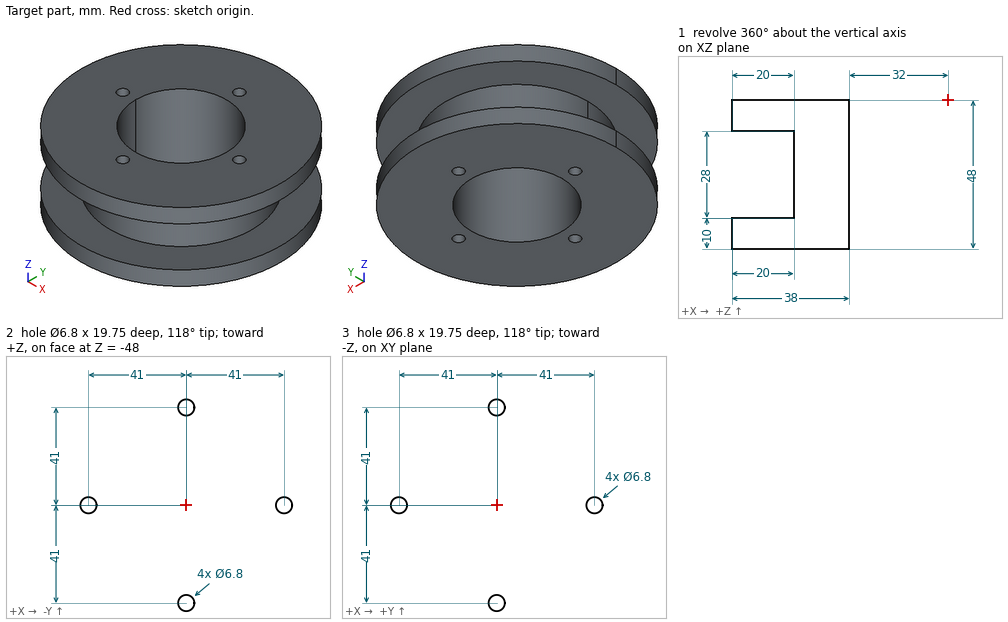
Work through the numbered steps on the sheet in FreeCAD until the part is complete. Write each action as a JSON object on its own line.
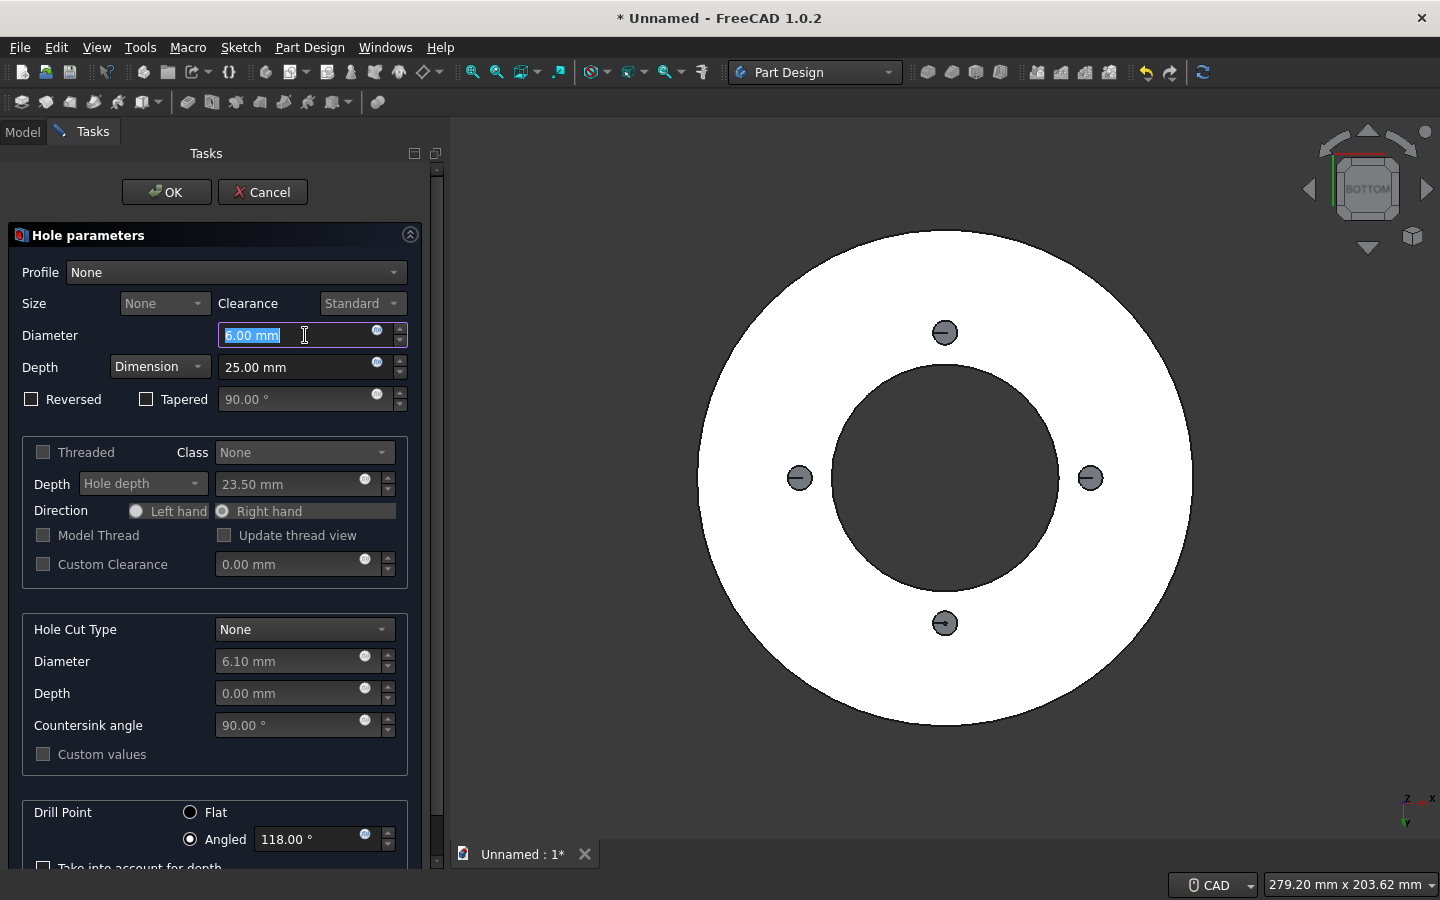
{"action": "type", "text": "6.8"}
{"action": "key", "text": "Tab"}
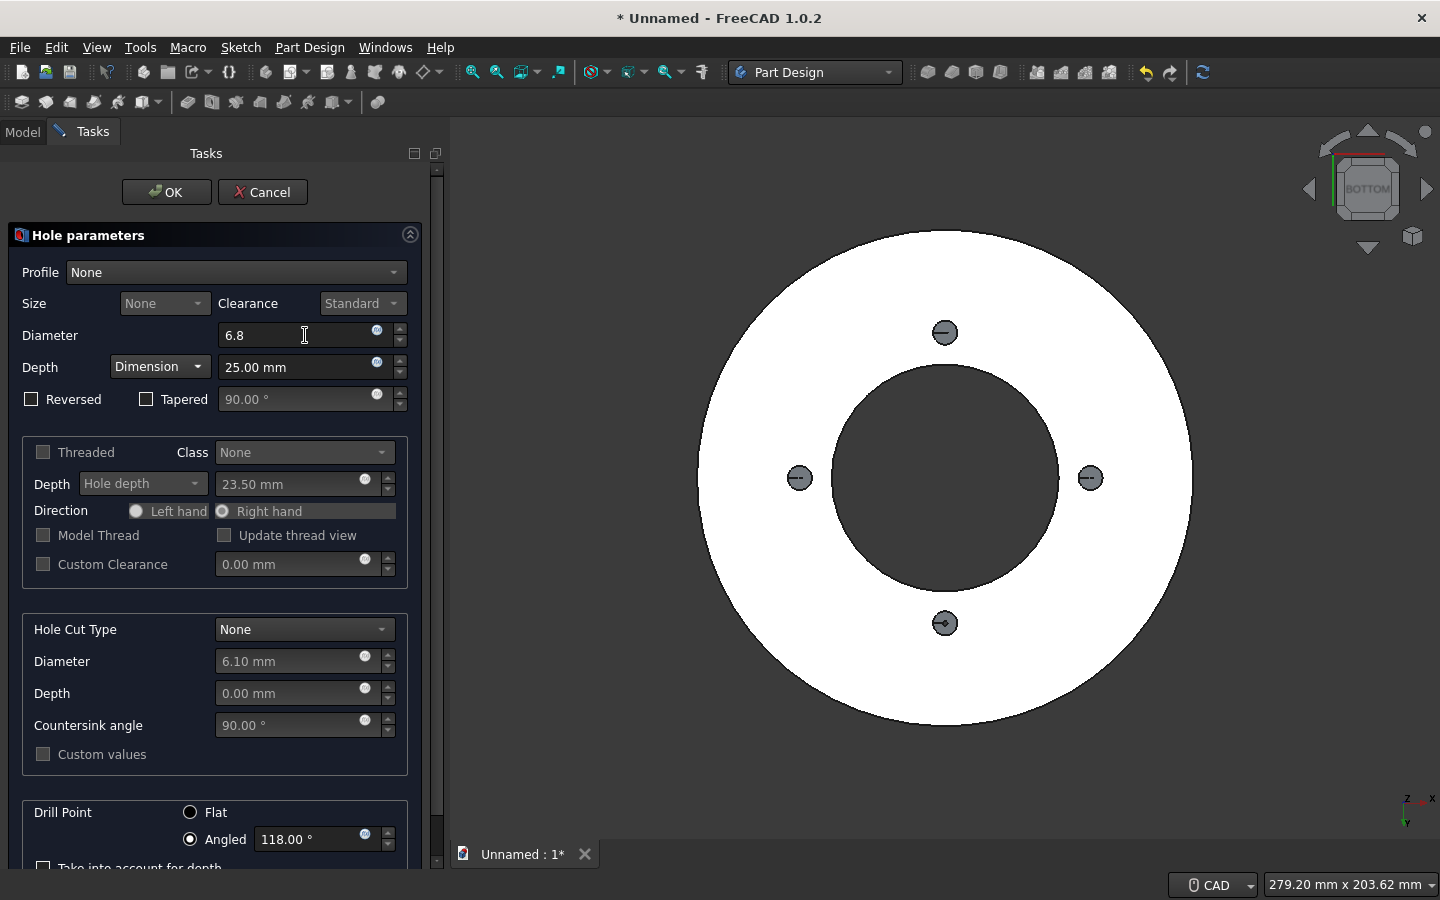
{"action": "triple_click", "coordinate": [305, 367]}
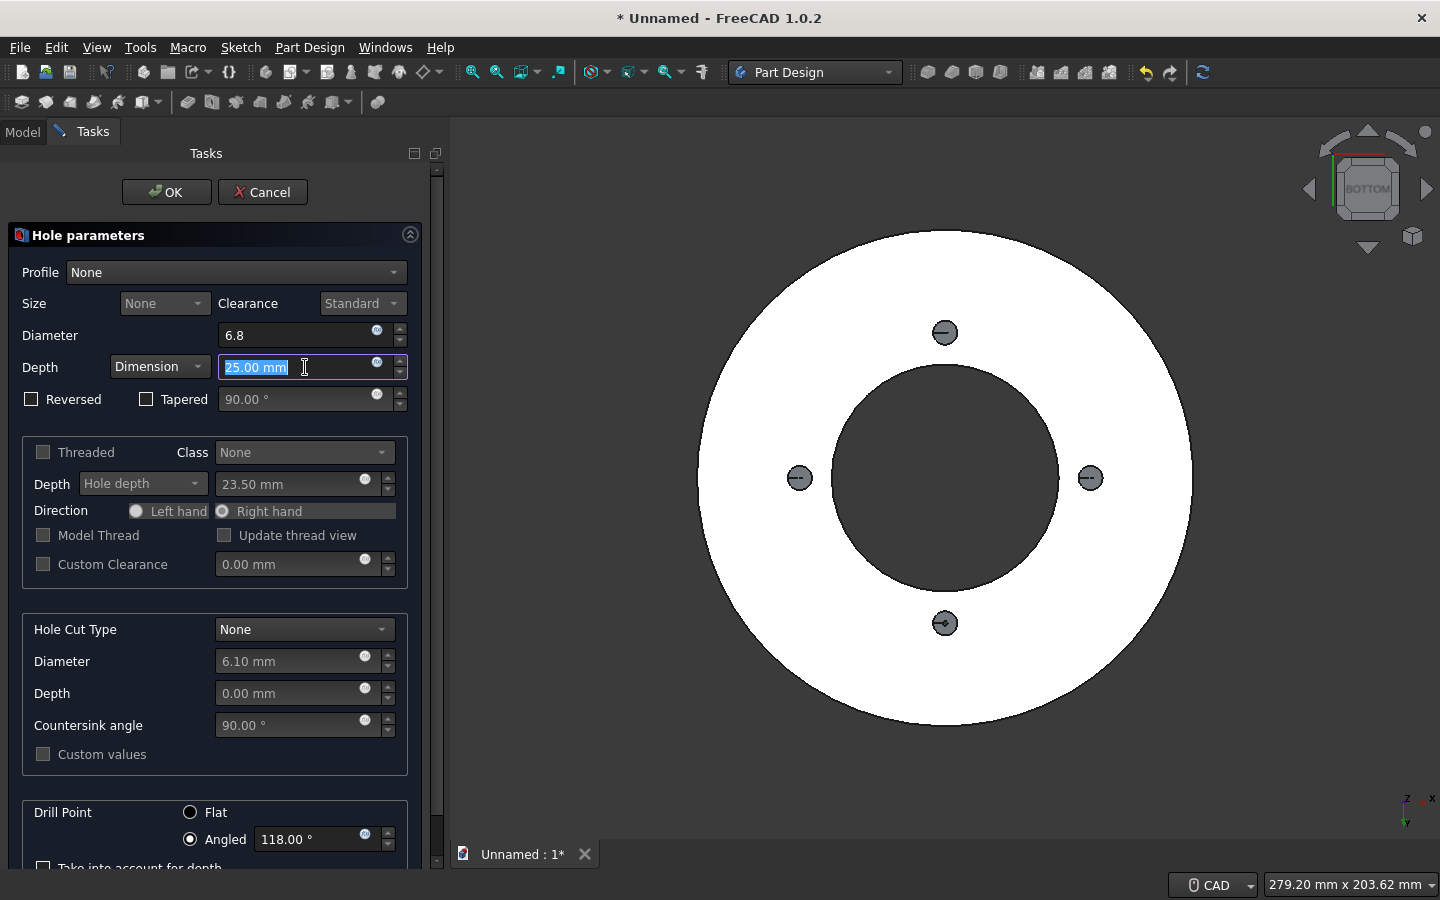
{"action": "type", "text": "19.75"}
{"action": "key", "text": "Tab"}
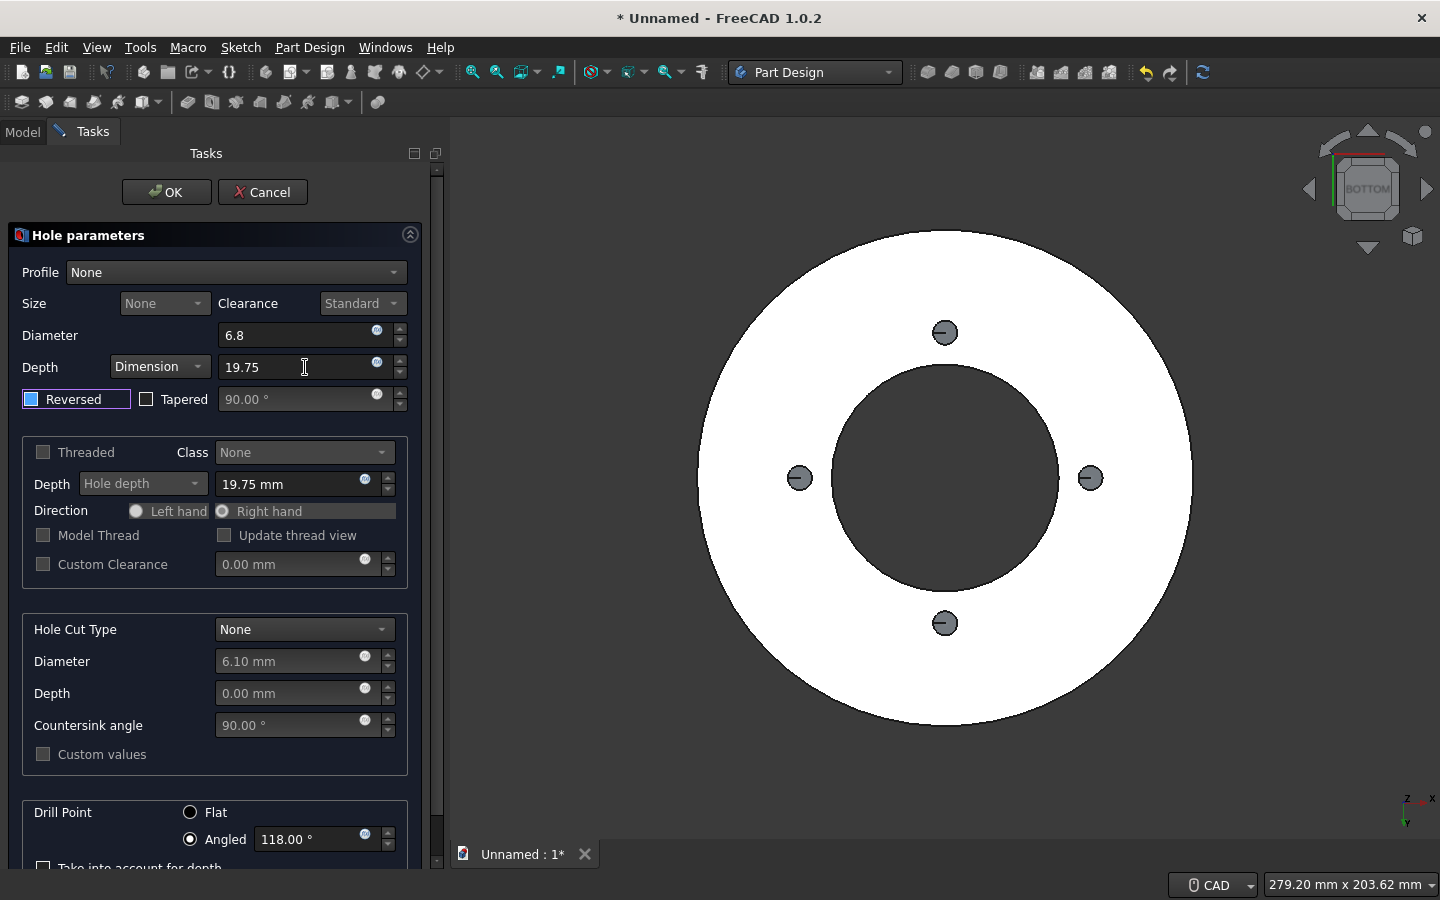
{"action": "left_click", "coordinate": [167, 192]}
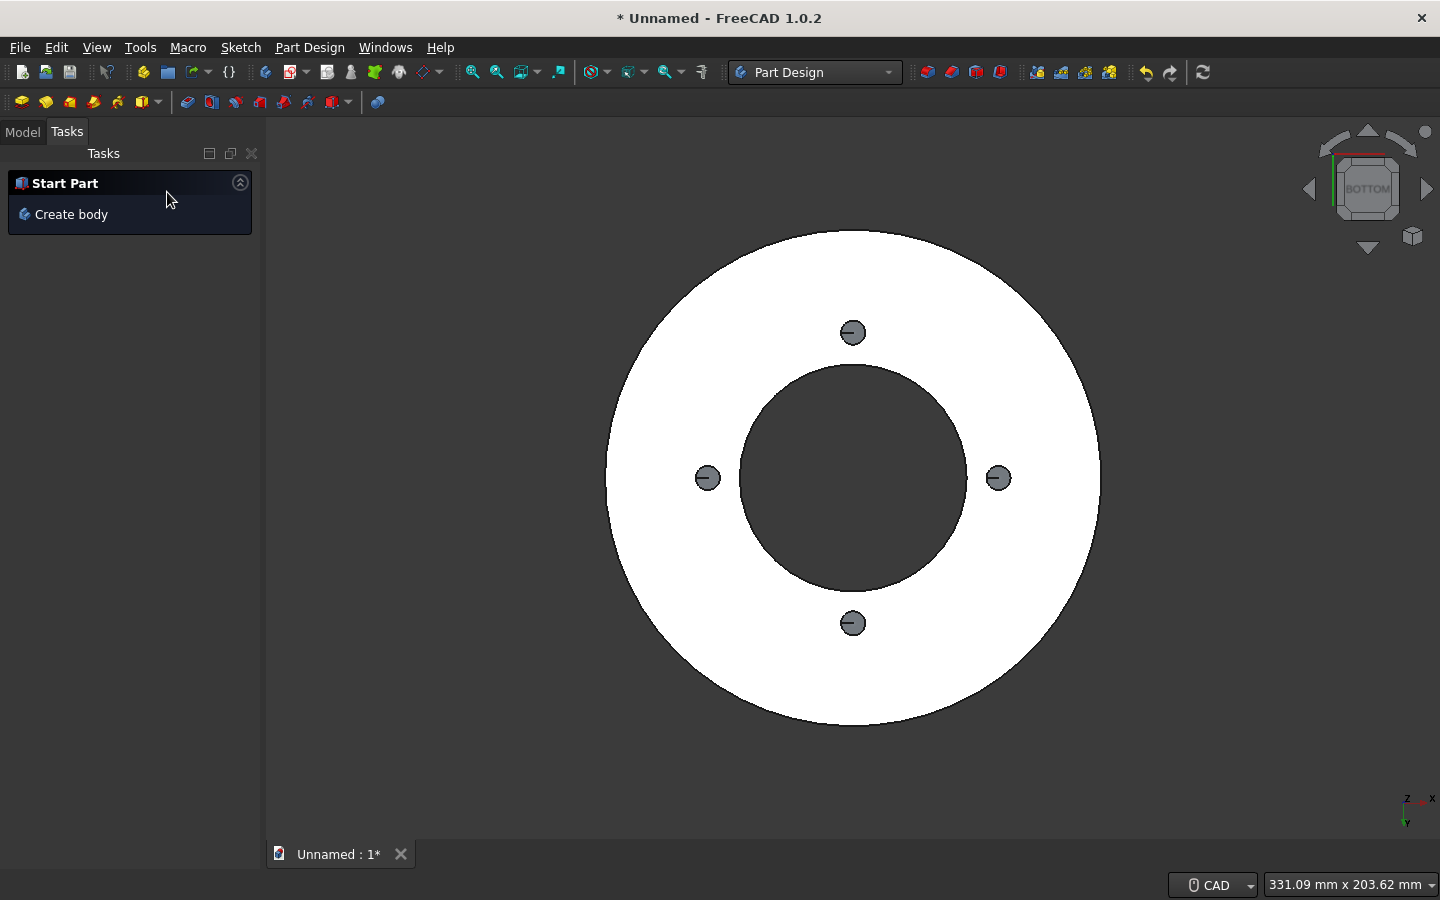
{"action": "key", "text": "0"}